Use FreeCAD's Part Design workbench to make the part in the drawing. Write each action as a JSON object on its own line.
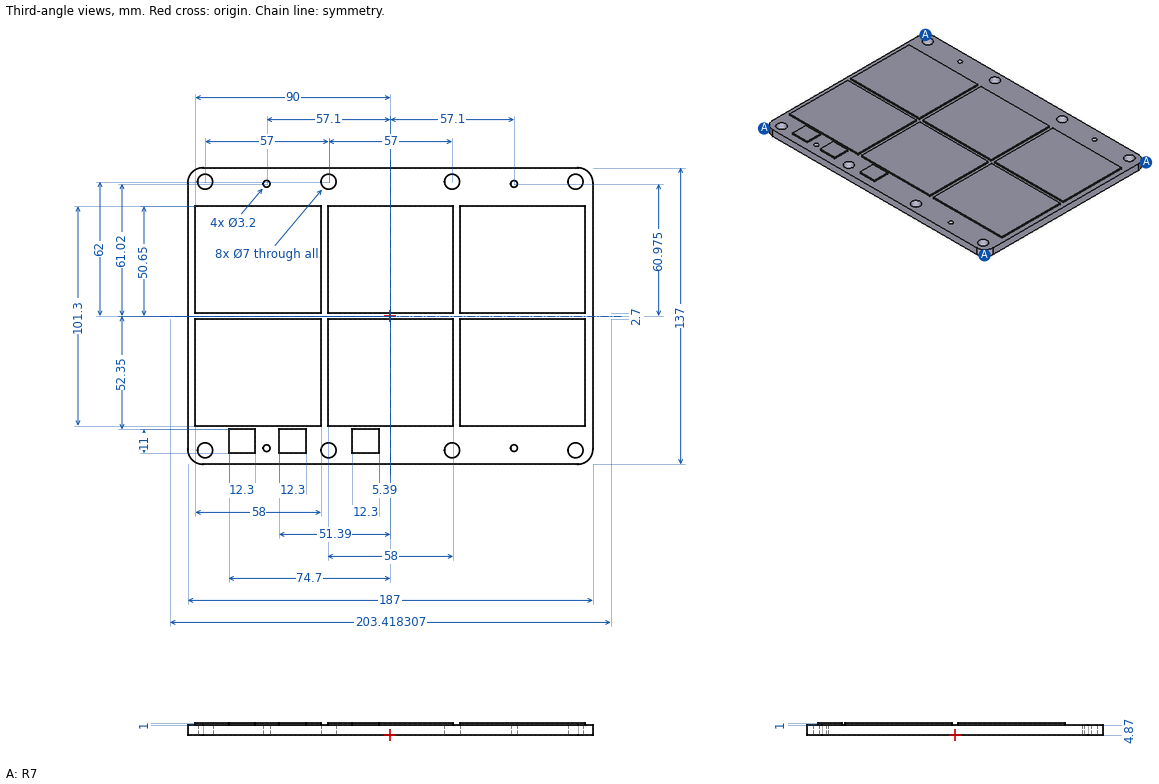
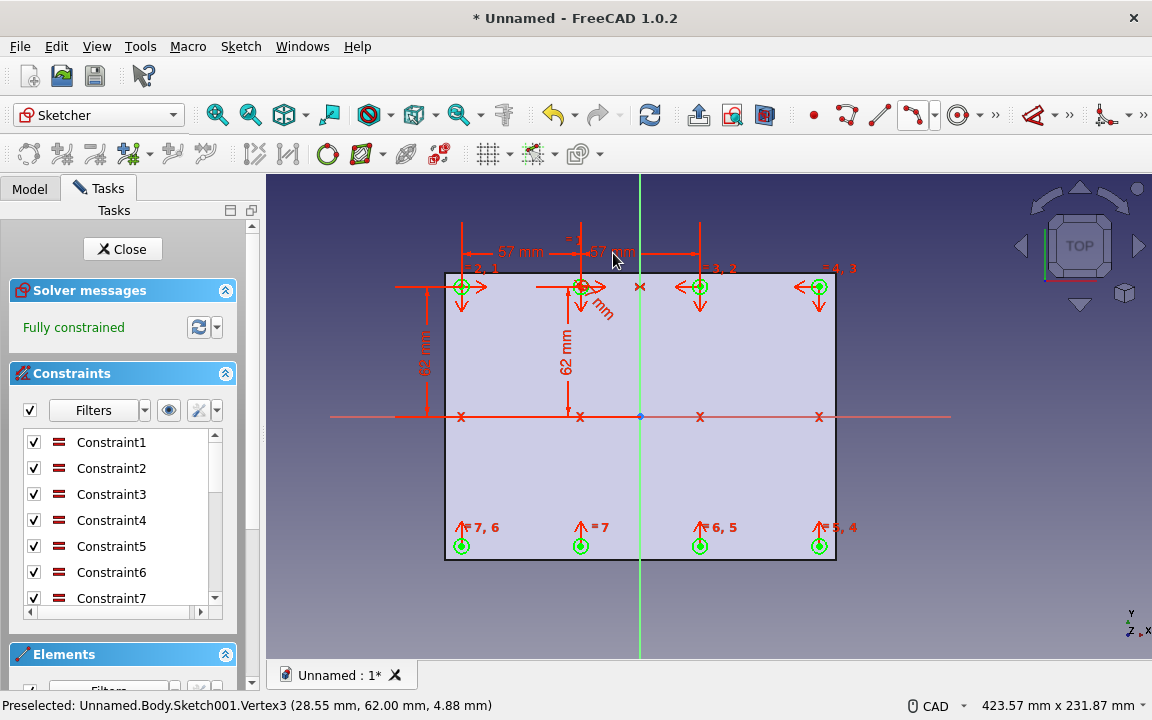
{"action": "left_click", "coordinate": [123, 249]}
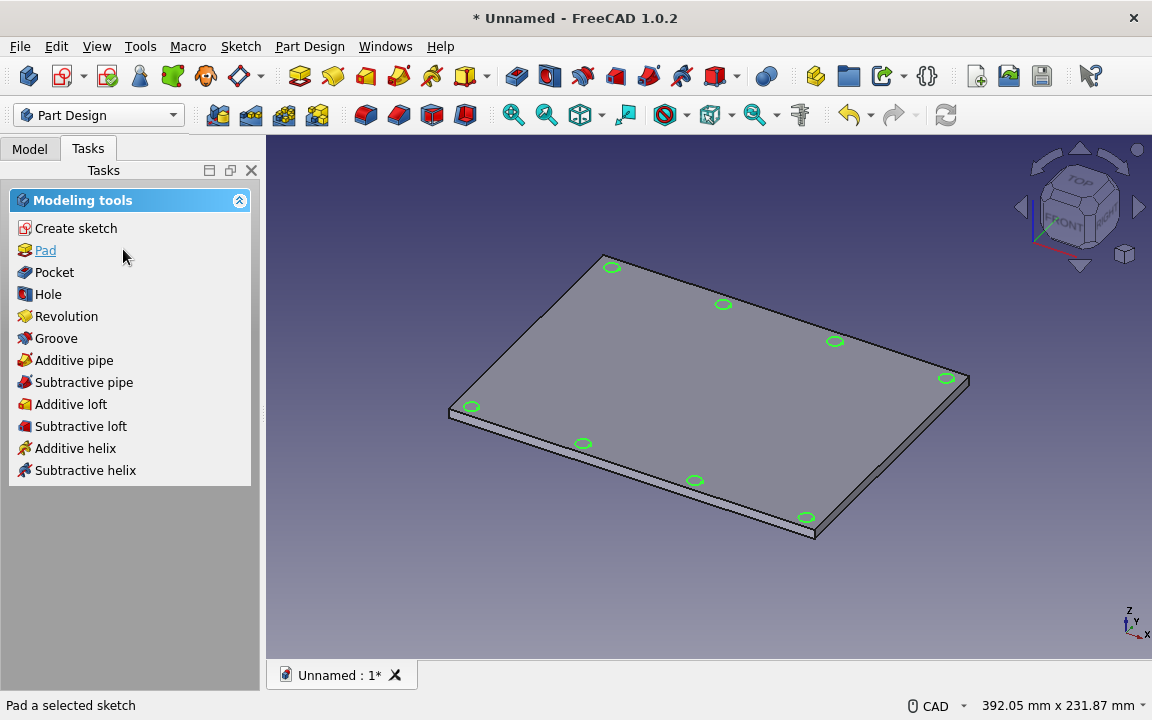
{"action": "left_click", "coordinate": [550, 76]}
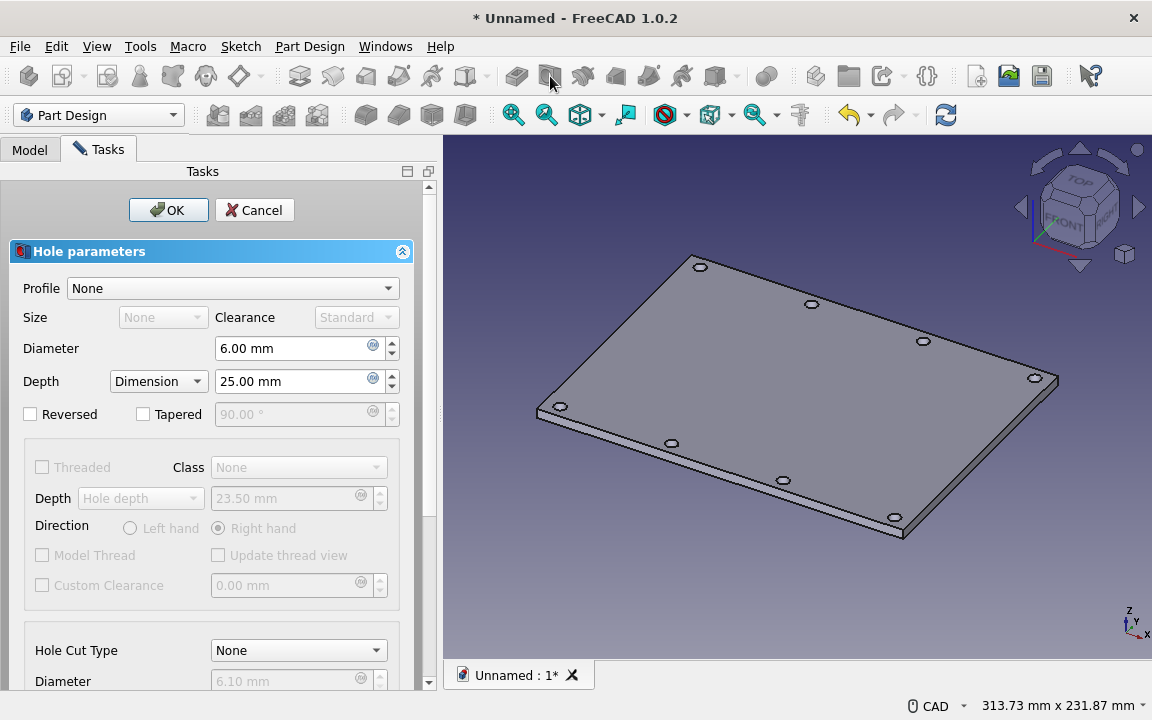
{"action": "triple_click", "coordinate": [300, 348]}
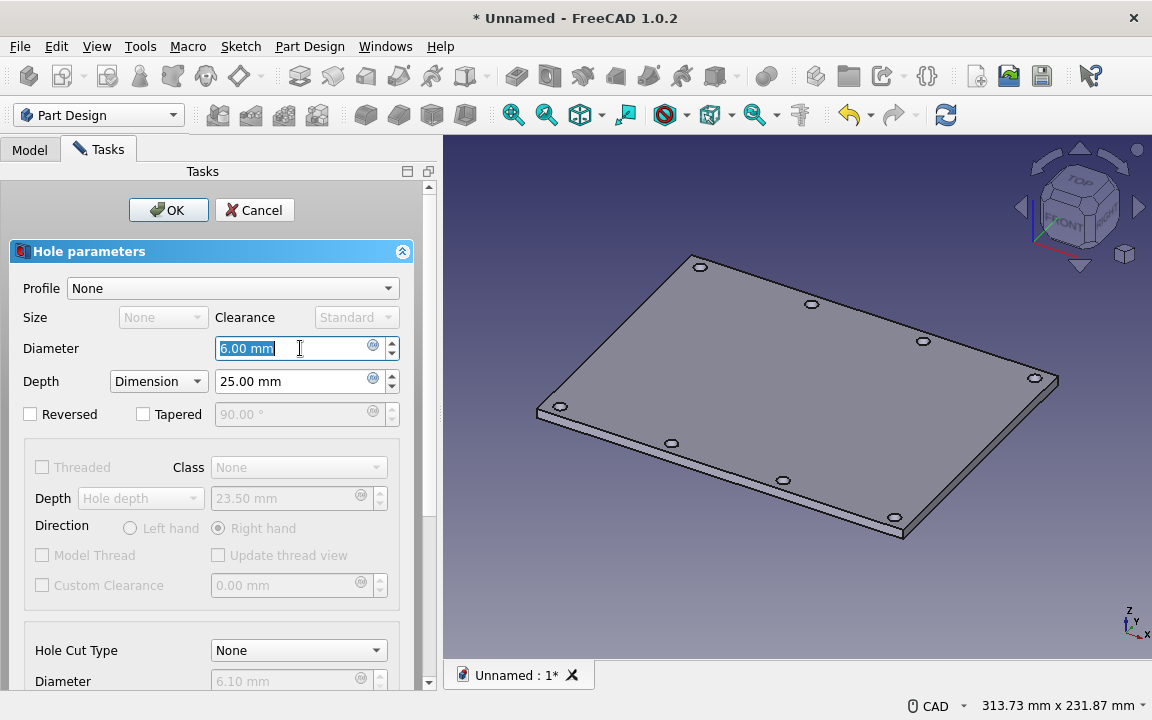
{"action": "type", "text": "7"}
{"action": "key", "text": "Tab"}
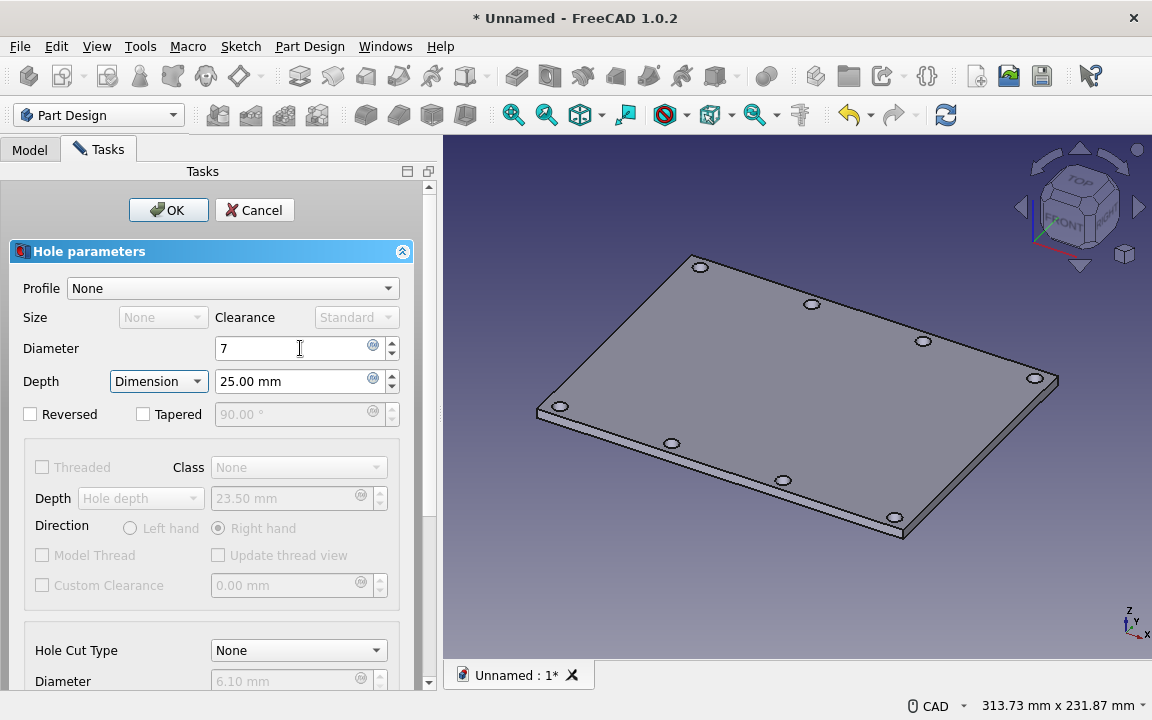
{"action": "left_click", "coordinate": [160, 382]}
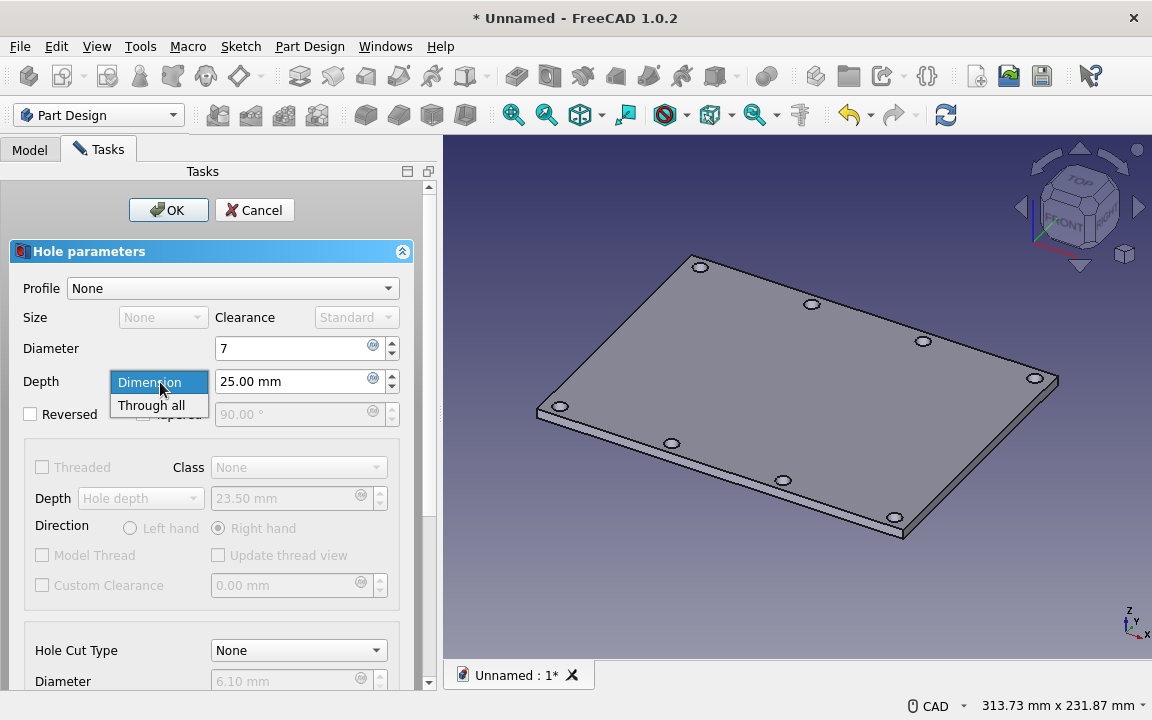
{"action": "left_click", "coordinate": [158, 406]}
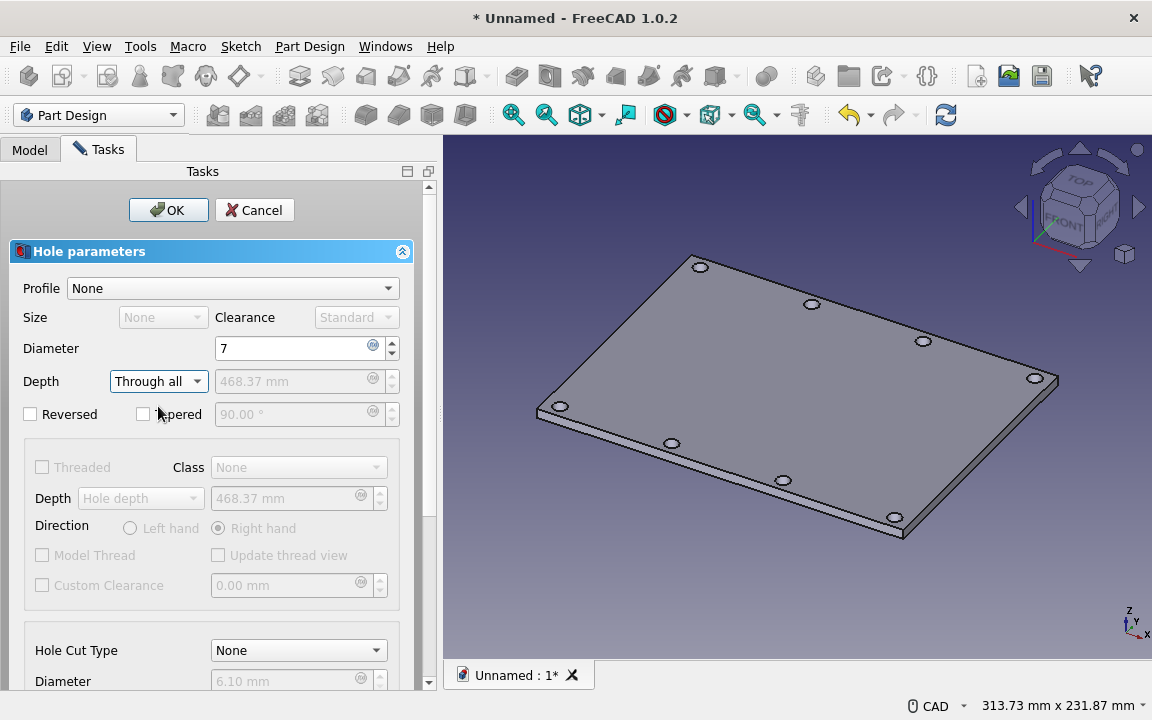
{"action": "left_click", "coordinate": [169, 210]}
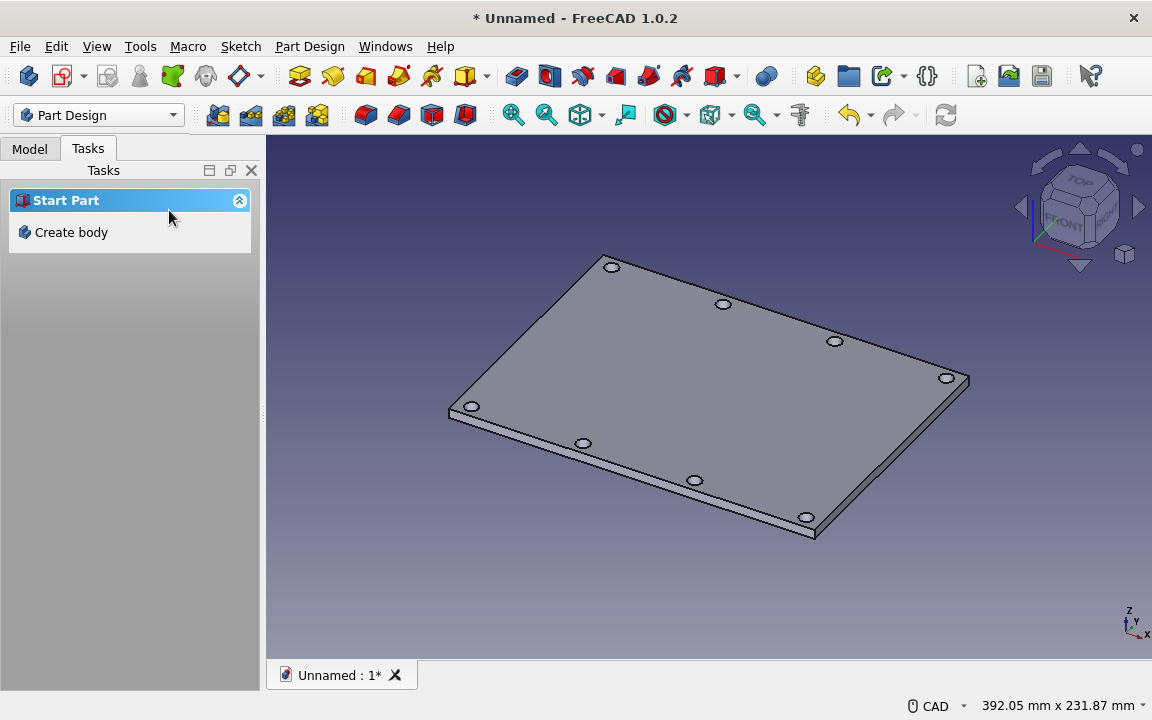
{"action": "left_click", "coordinate": [709, 391]}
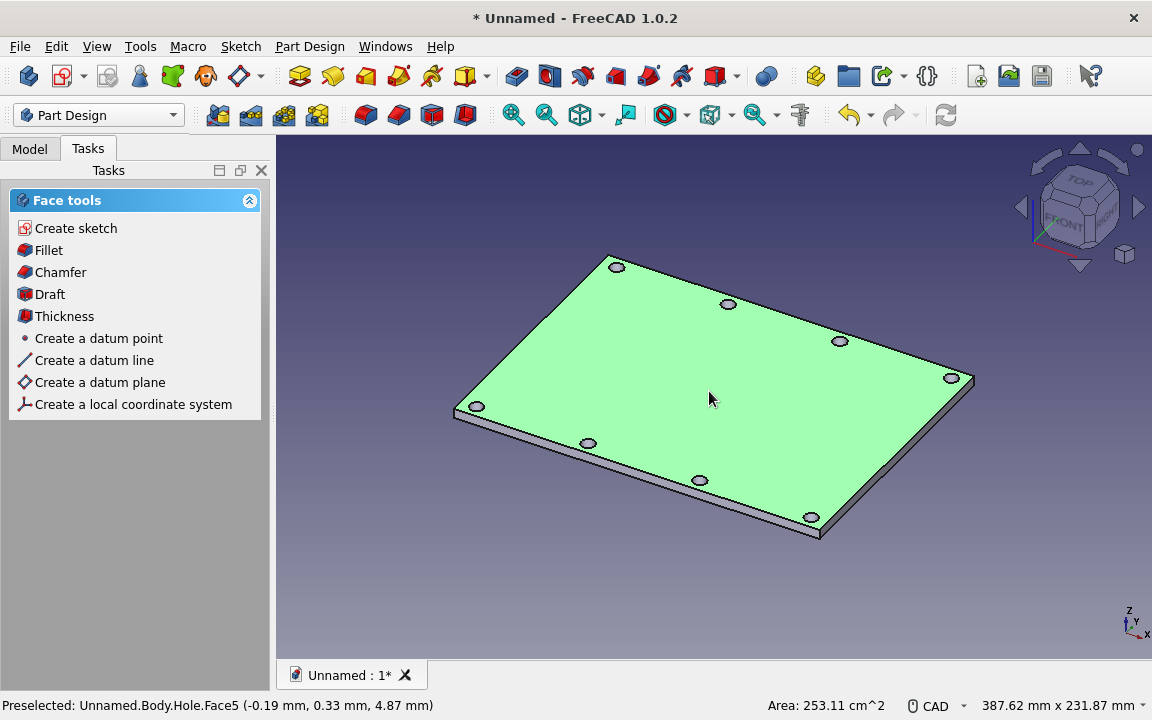
{"action": "left_click", "coordinate": [62, 76]}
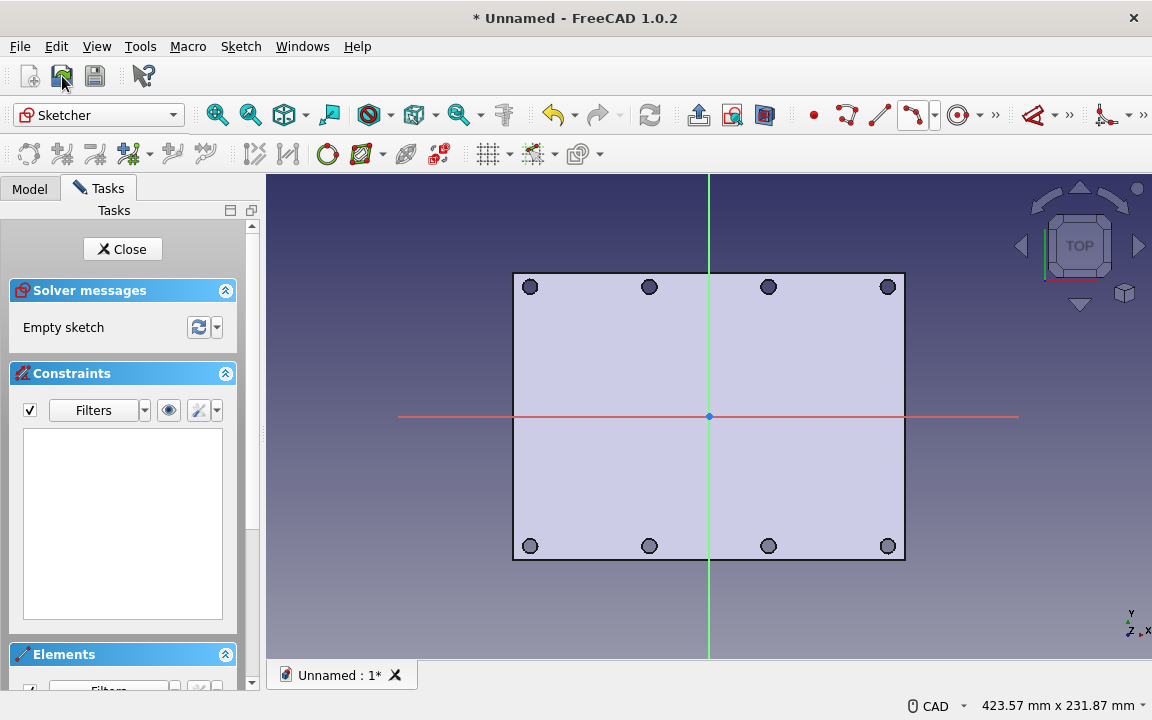
{"action": "left_click", "coordinate": [958, 116]}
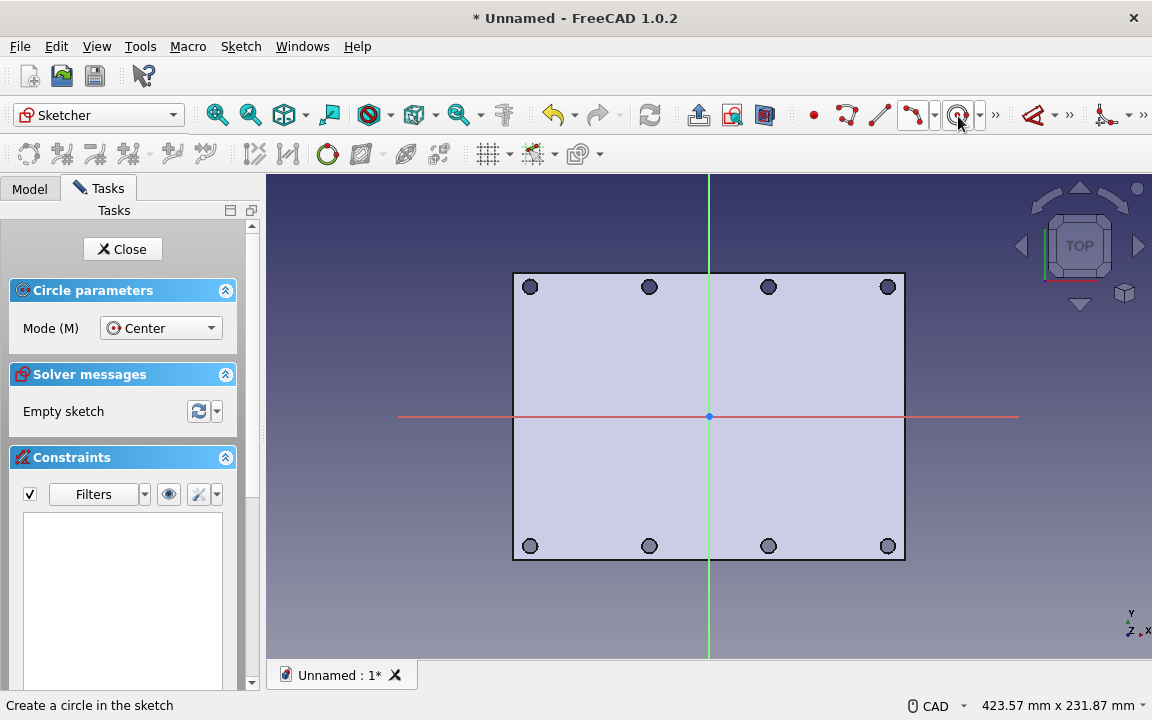
{"action": "scroll", "coordinate": [590, 289], "scroll_direction": "up", "scroll_amount": 10}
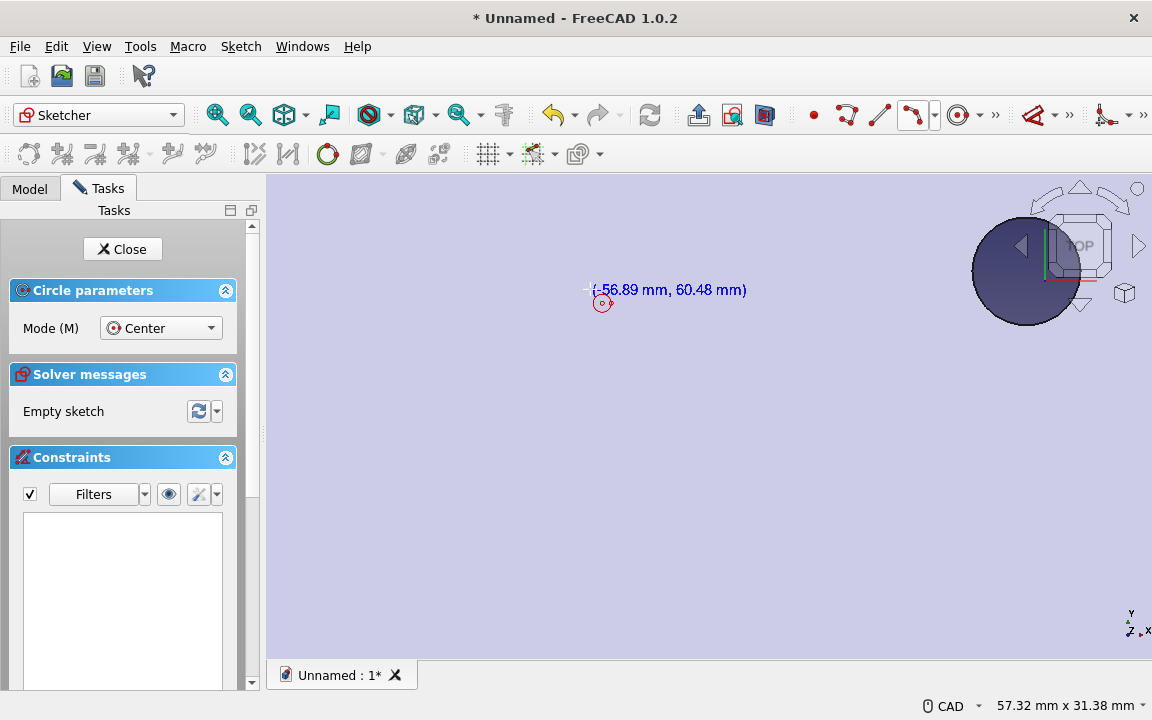
{"action": "scroll", "coordinate": [477, 255], "scroll_direction": "down", "scroll_amount": 9}